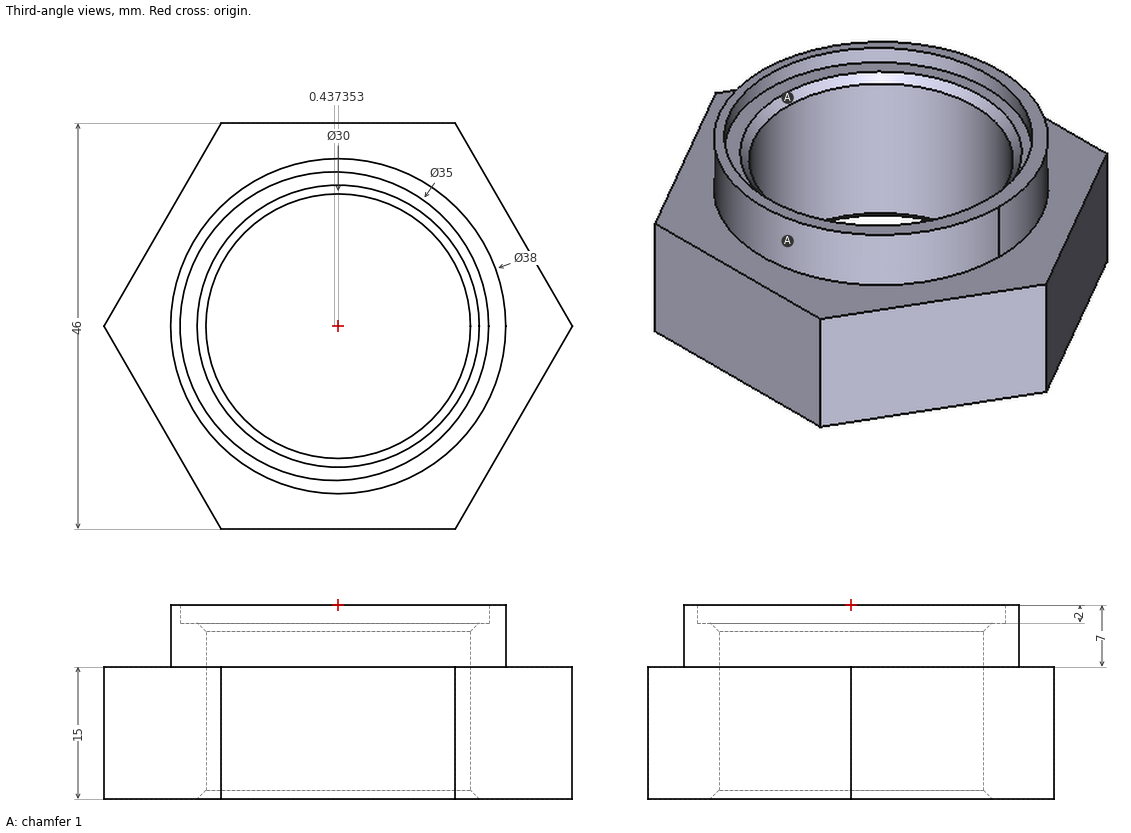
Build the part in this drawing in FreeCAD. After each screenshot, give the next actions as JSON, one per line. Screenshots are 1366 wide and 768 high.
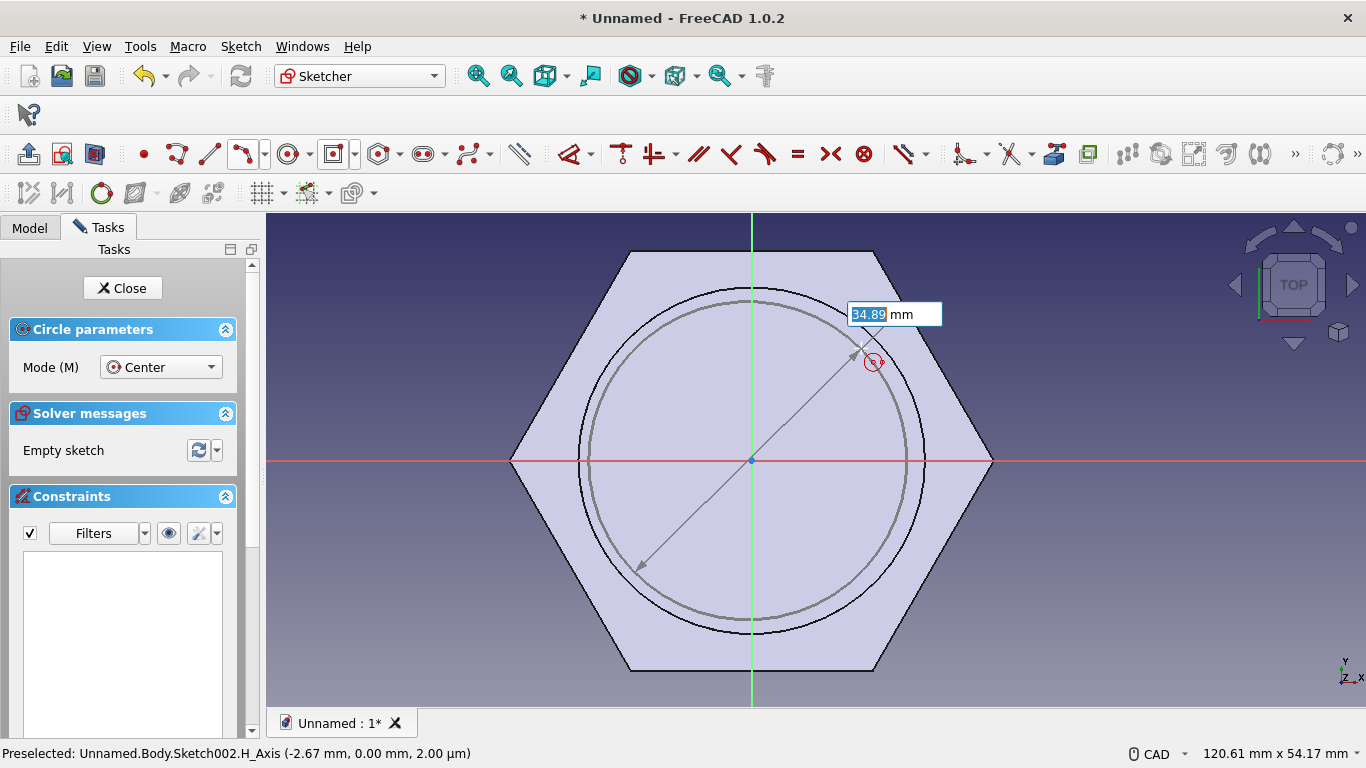
{"action": "type", "text": "35"}
{"action": "key", "text": "Return"}
{"action": "key", "text": "Escape"}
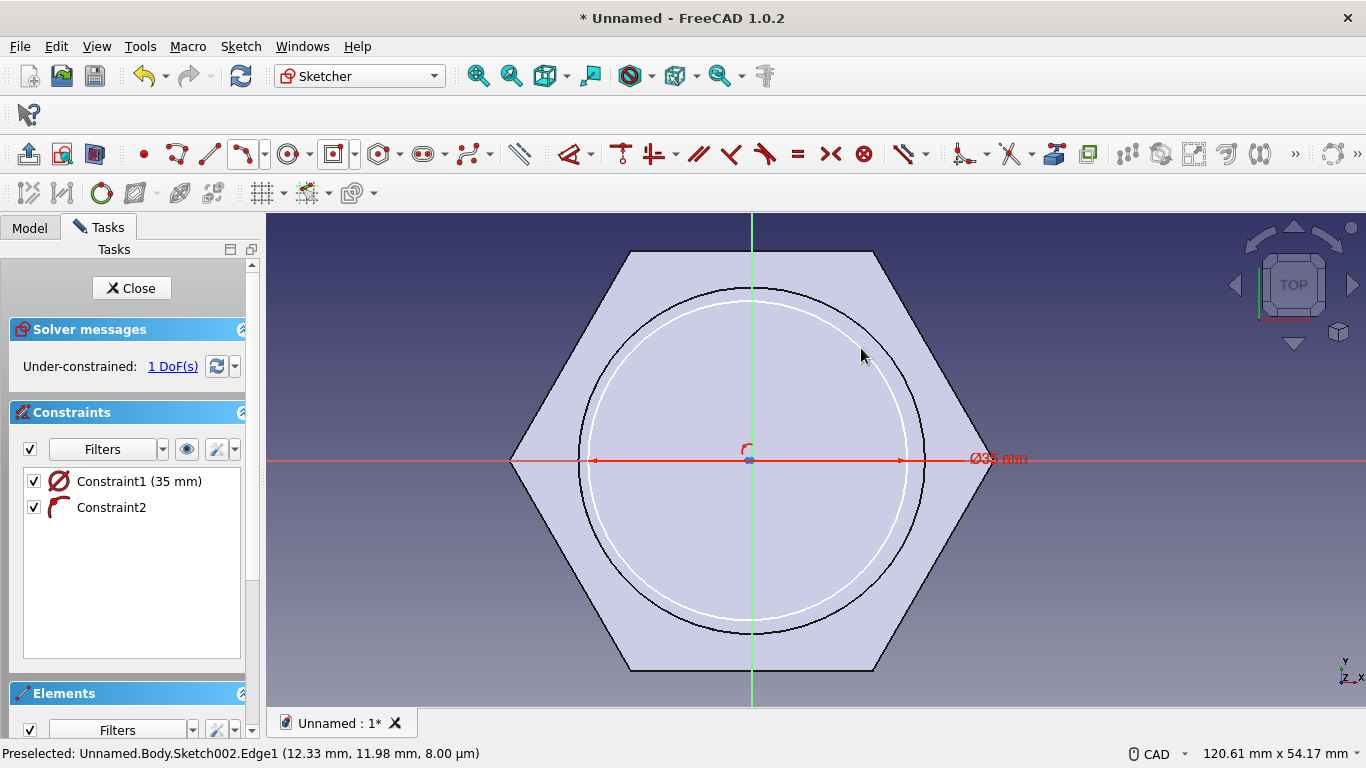
{"action": "left_click", "coordinate": [568, 154]}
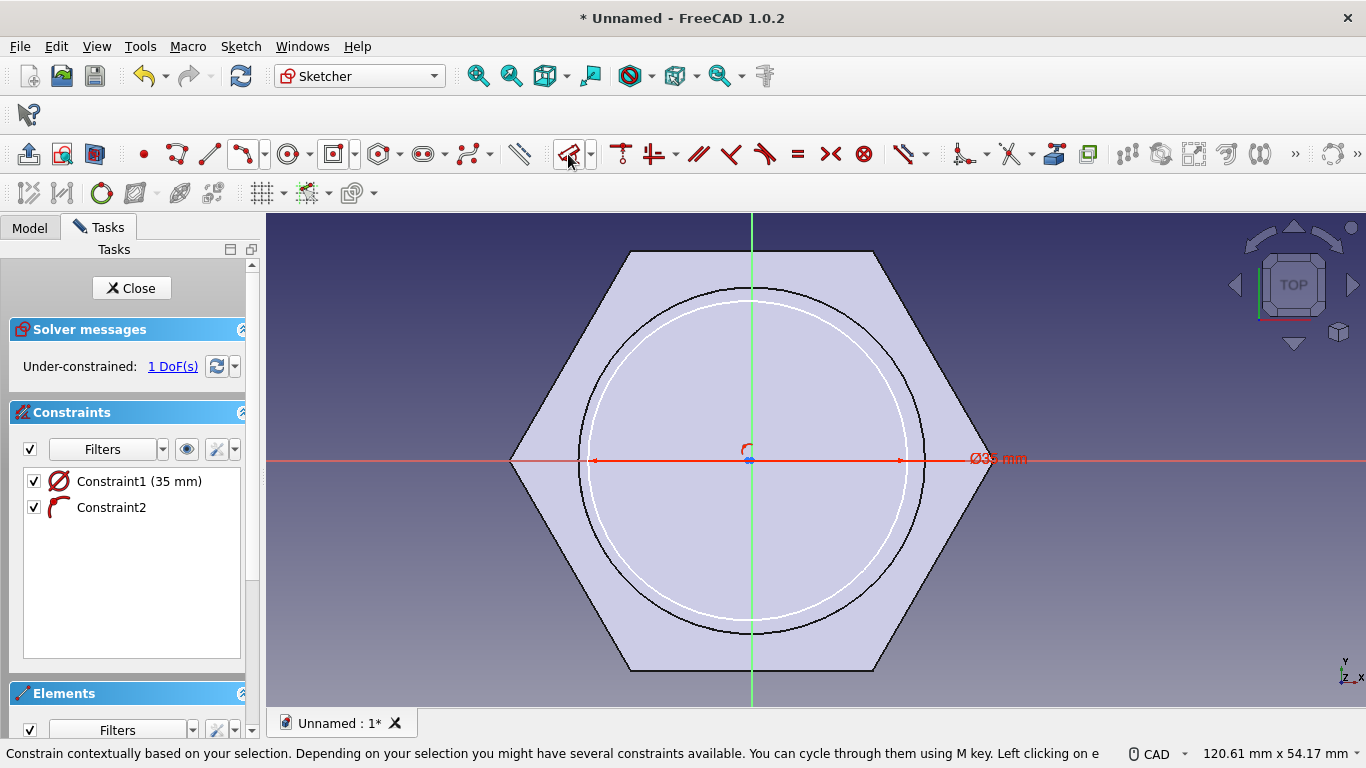
{"action": "scroll", "coordinate": [748, 461], "scroll_direction": "up", "scroll_amount": 12}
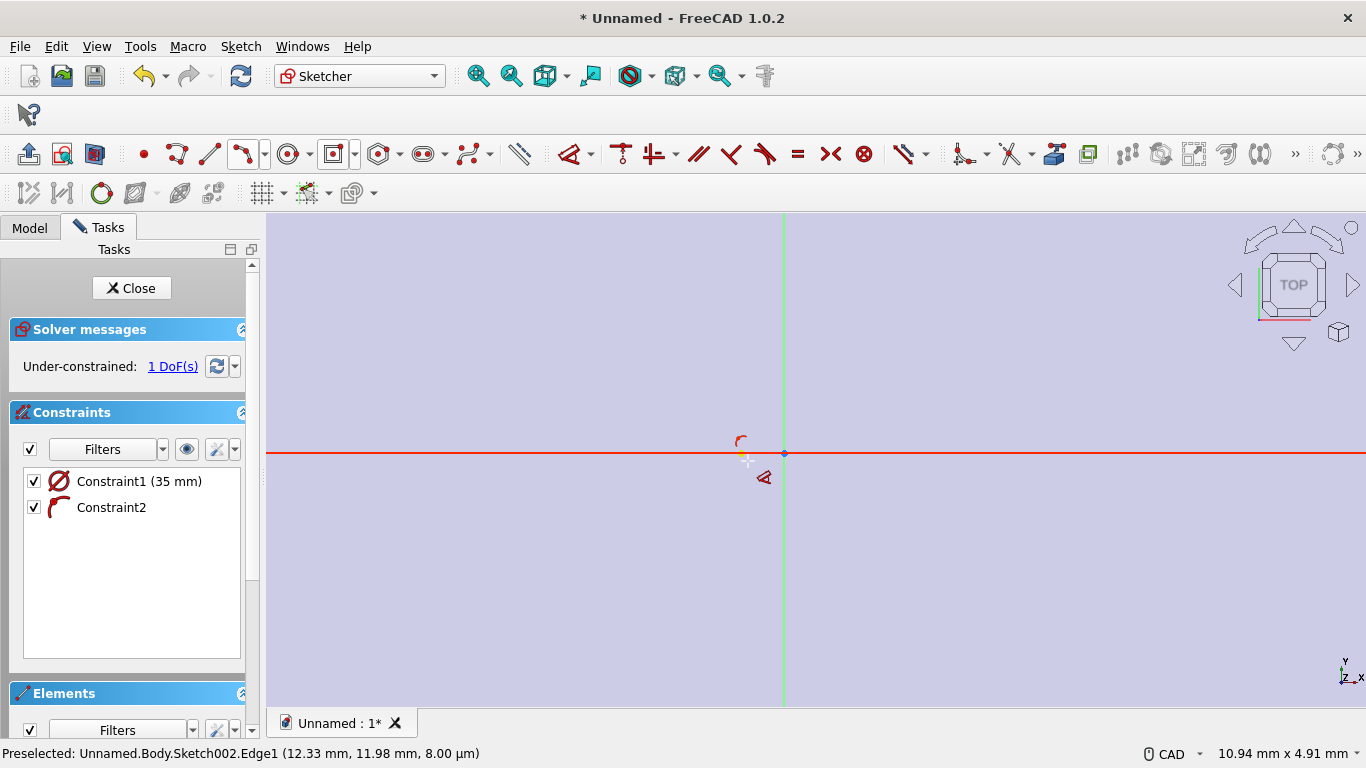
{"action": "left_click", "coordinate": [741, 453]}
{"action": "left_click", "coordinate": [763, 487]}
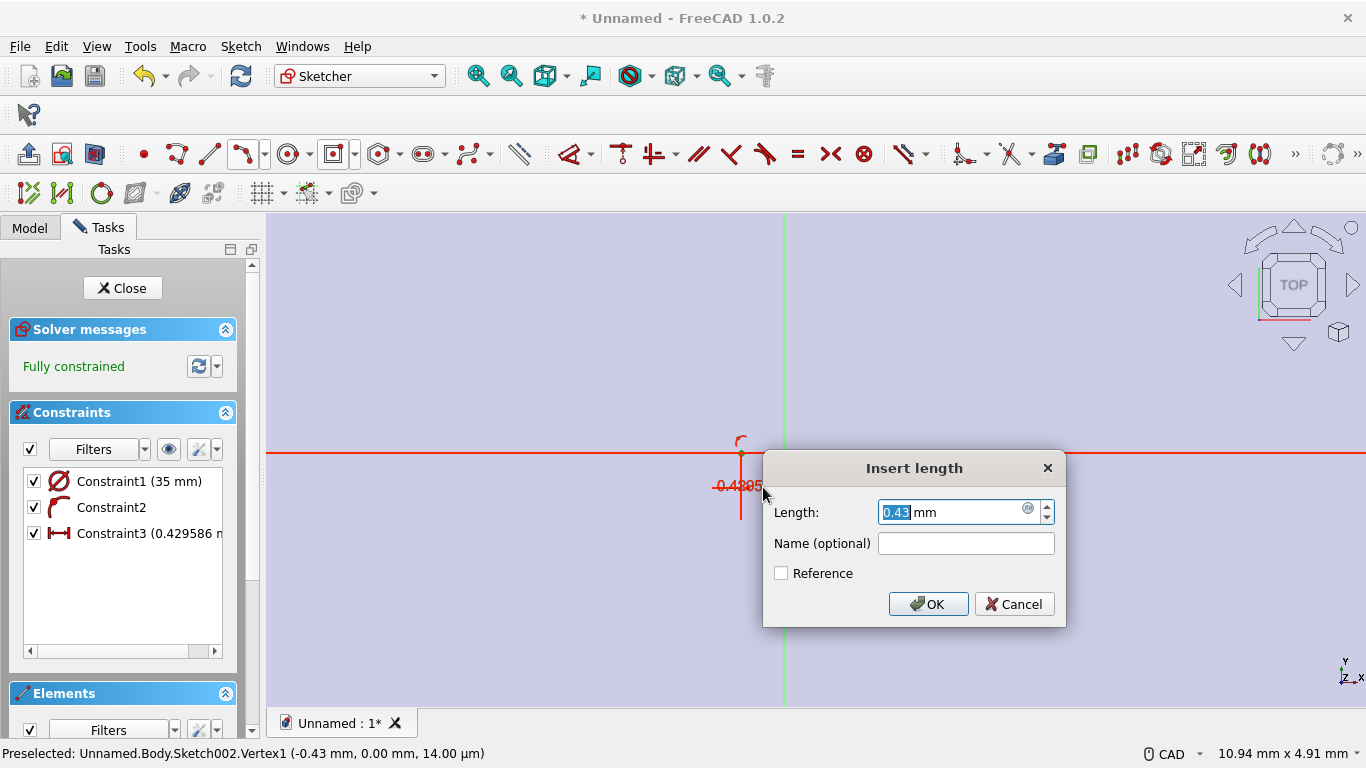
{"action": "type", "text": "0.437353"}
{"action": "key", "text": "Return"}
{"action": "key", "text": "Escape"}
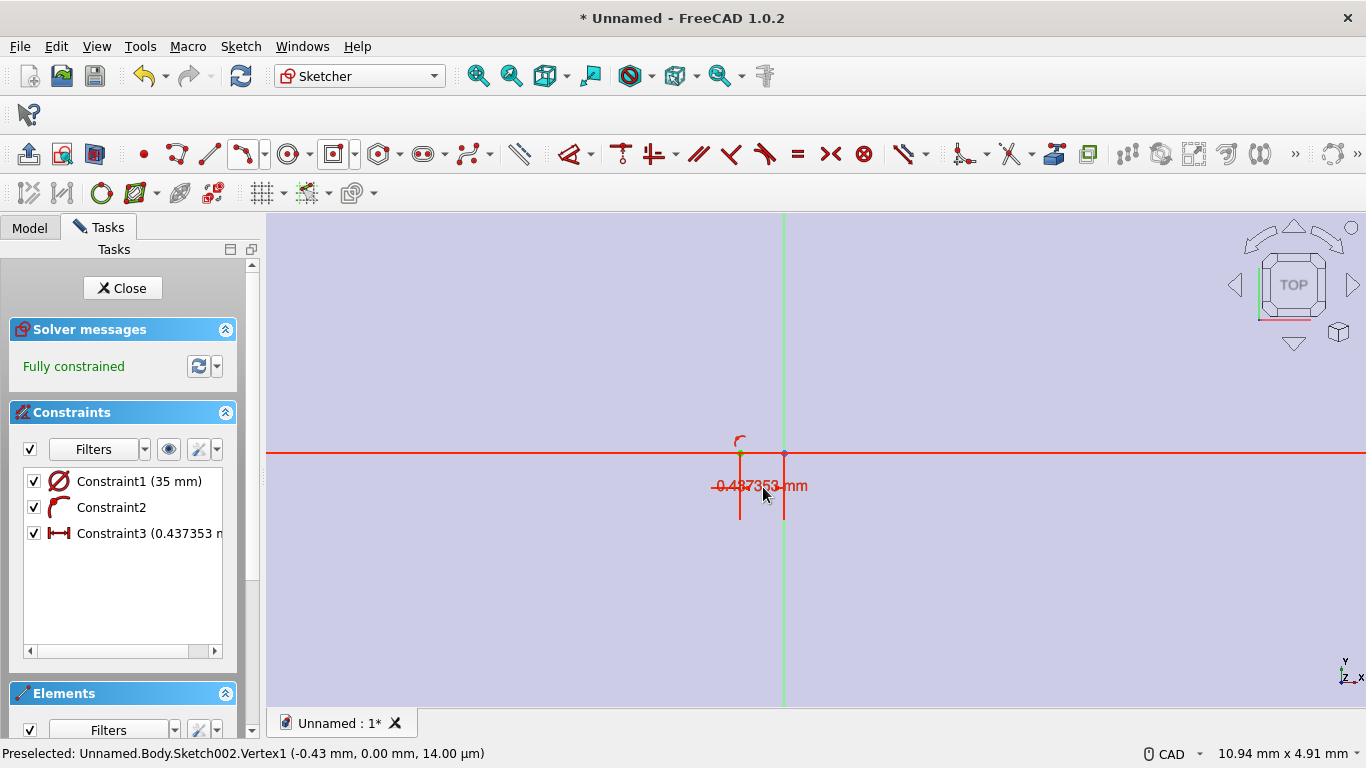
{"action": "left_click", "coordinate": [123, 288]}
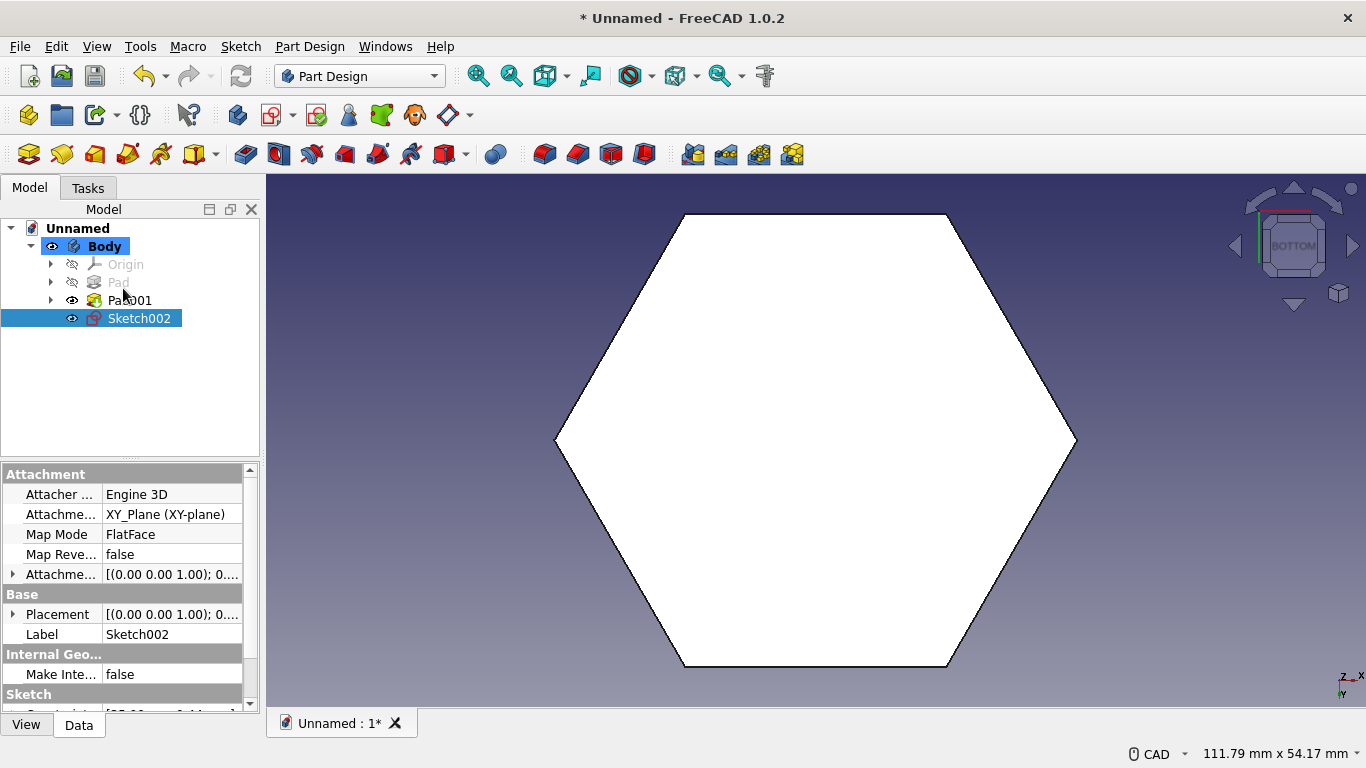
{"action": "left_click", "coordinate": [246, 154]}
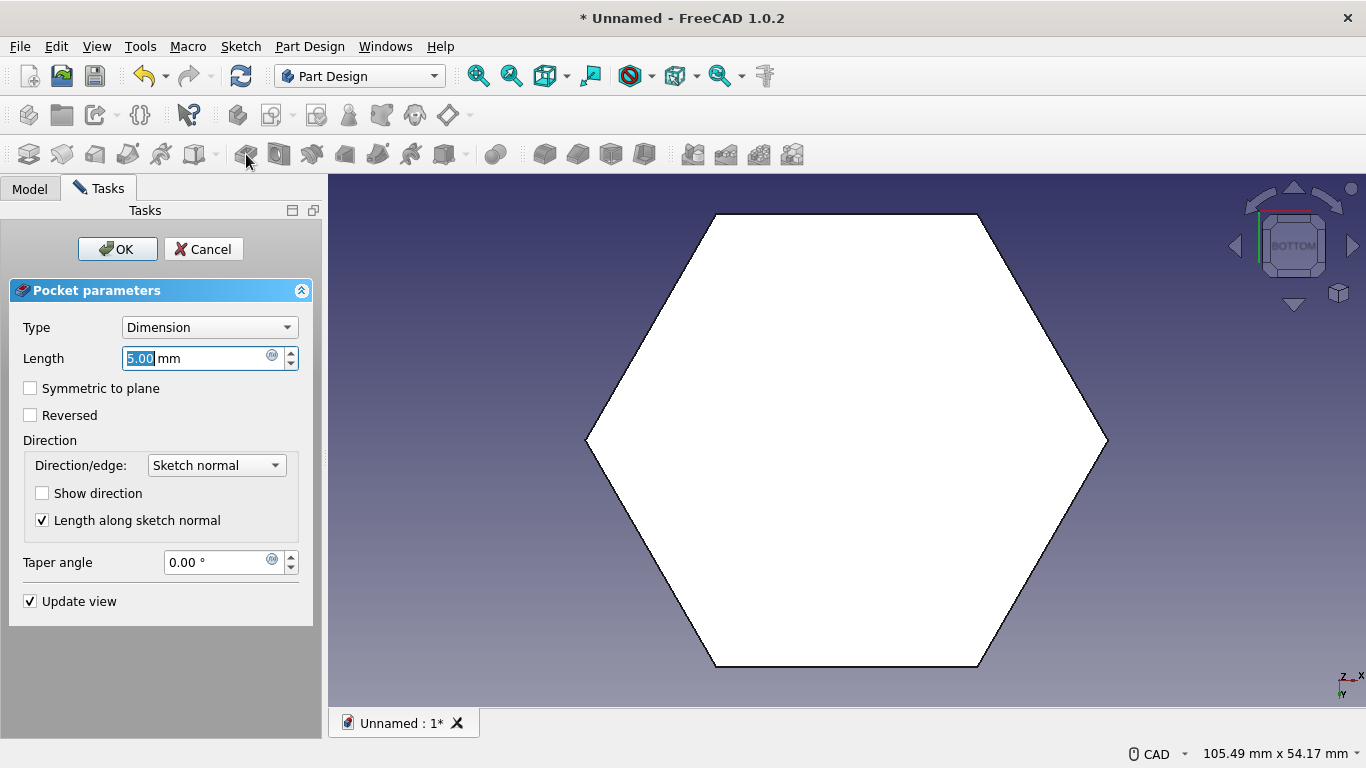
{"action": "type", "text": "2"}
{"action": "key", "text": "Tab"}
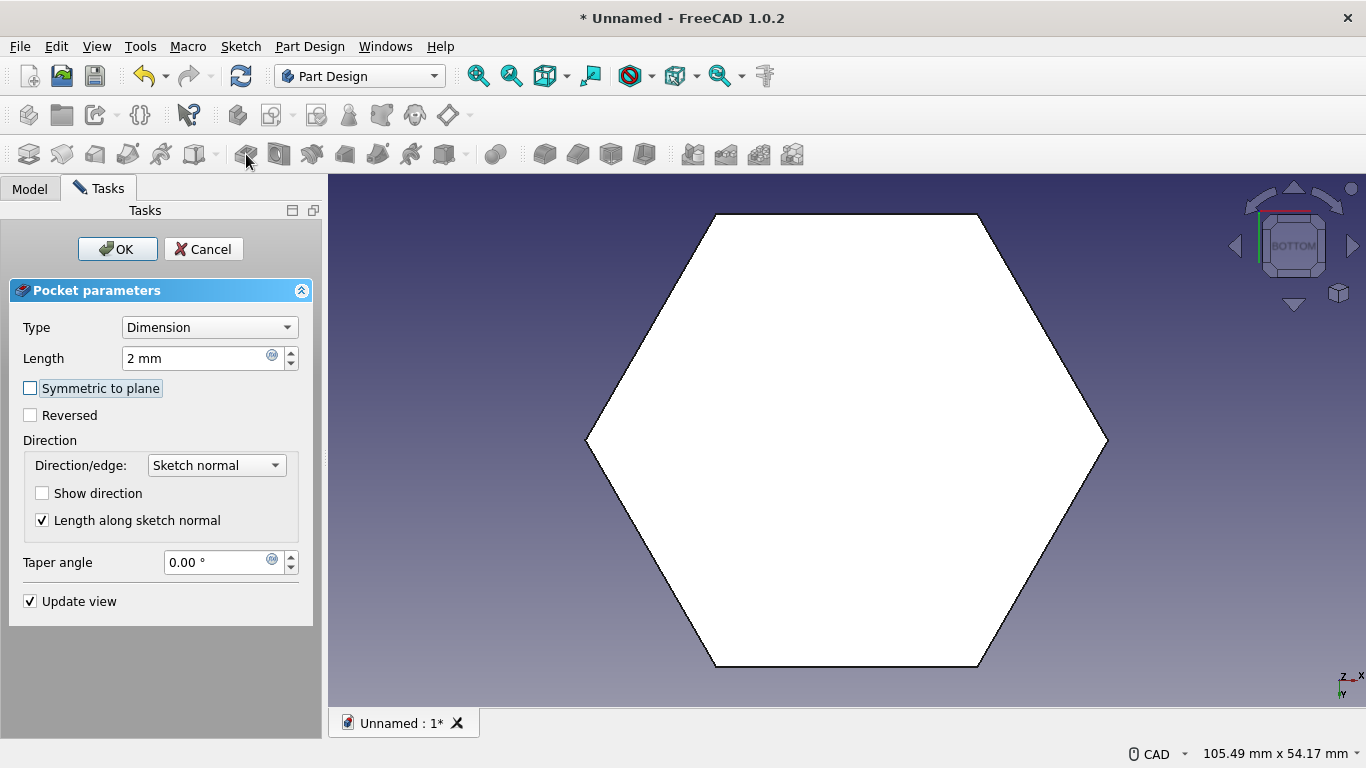
{"action": "left_click", "coordinate": [118, 249]}